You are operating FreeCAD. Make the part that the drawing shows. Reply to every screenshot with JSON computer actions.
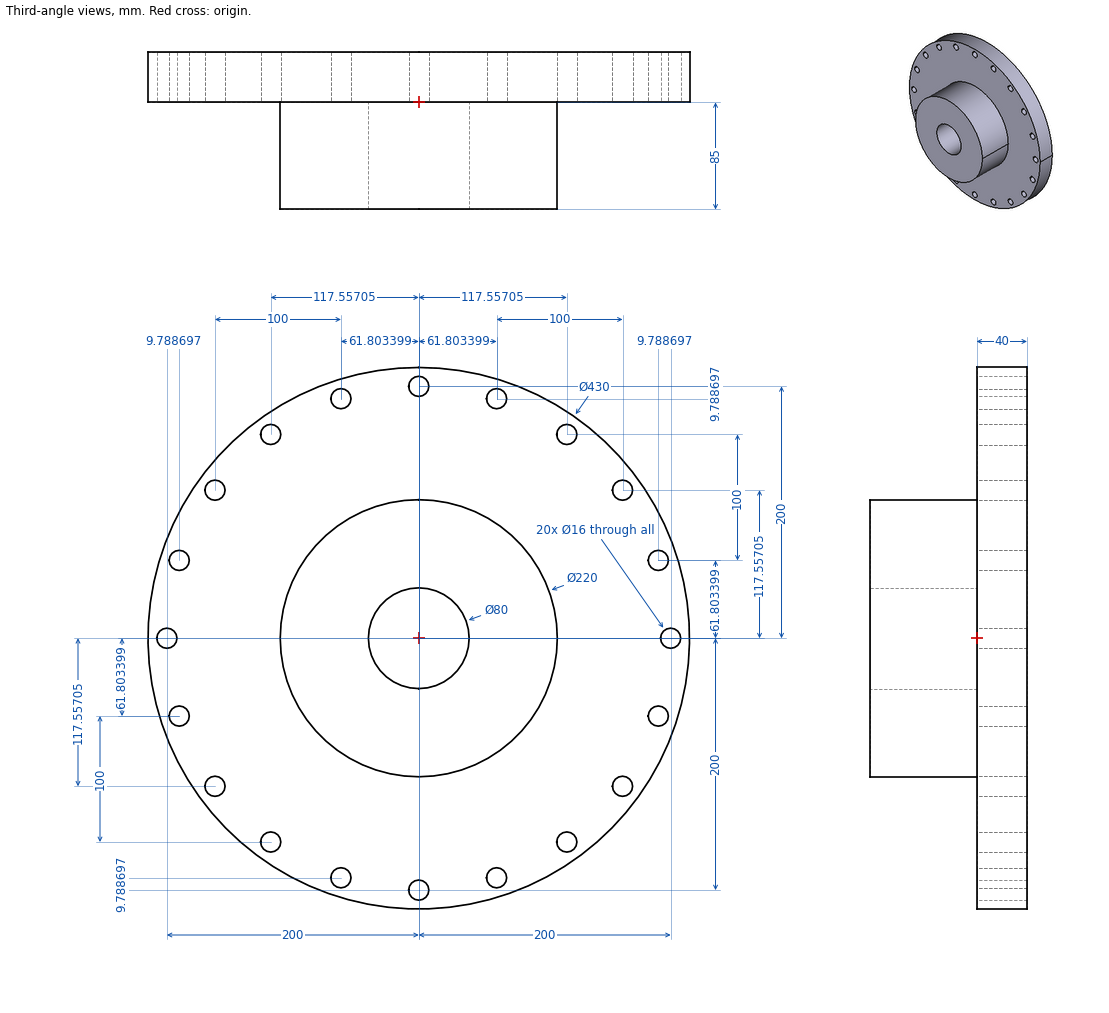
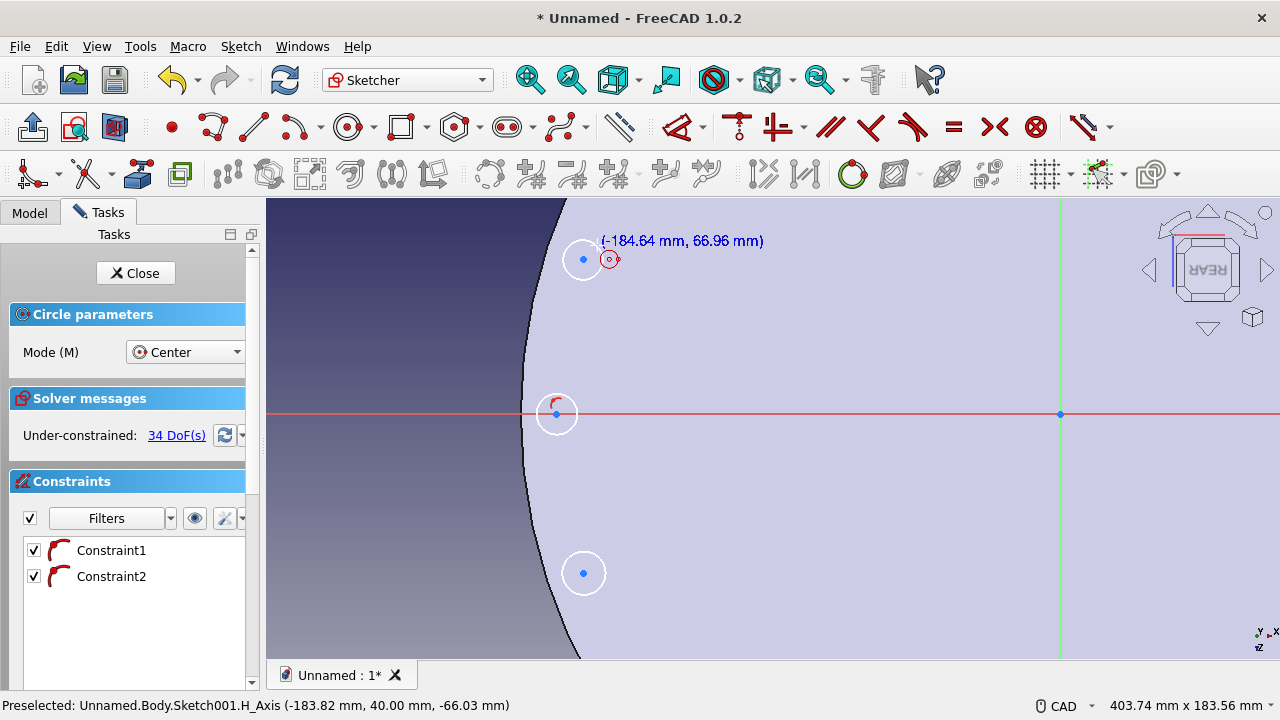
{"action": "scroll", "coordinate": [551, 435], "scroll_direction": "down", "scroll_amount": 6}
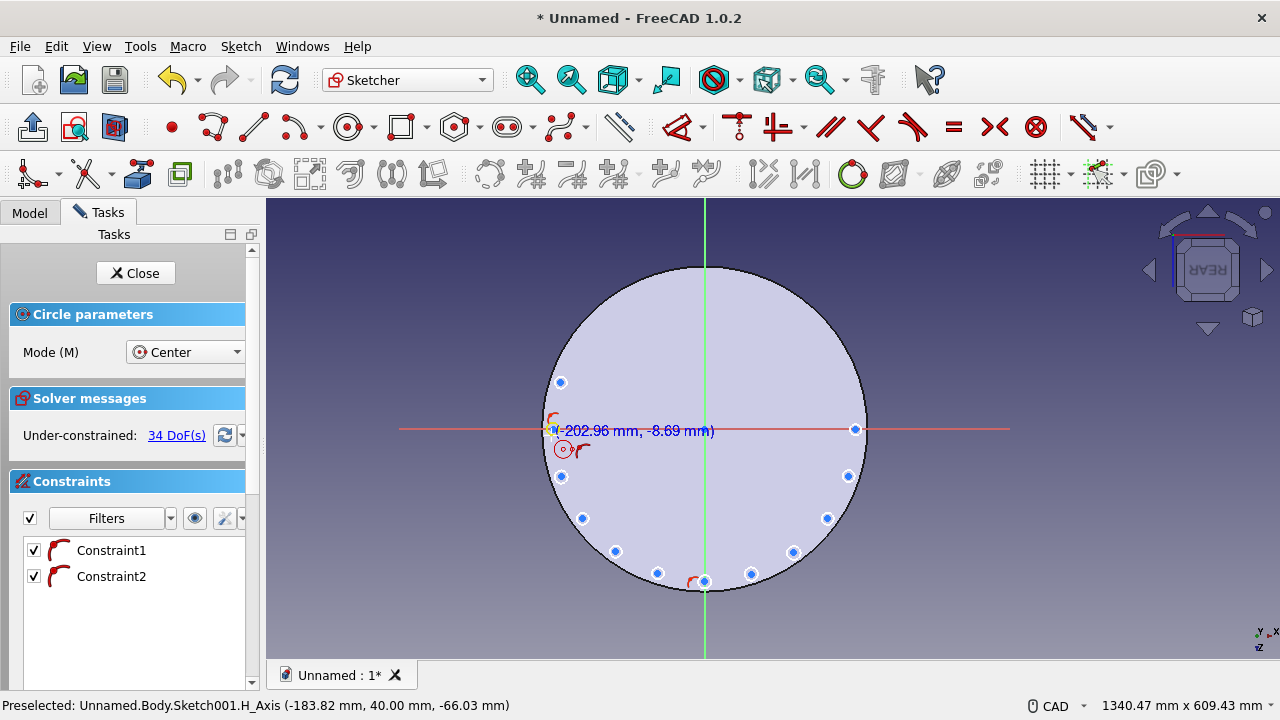
{"action": "scroll", "coordinate": [582, 340], "scroll_direction": "up", "scroll_amount": 7}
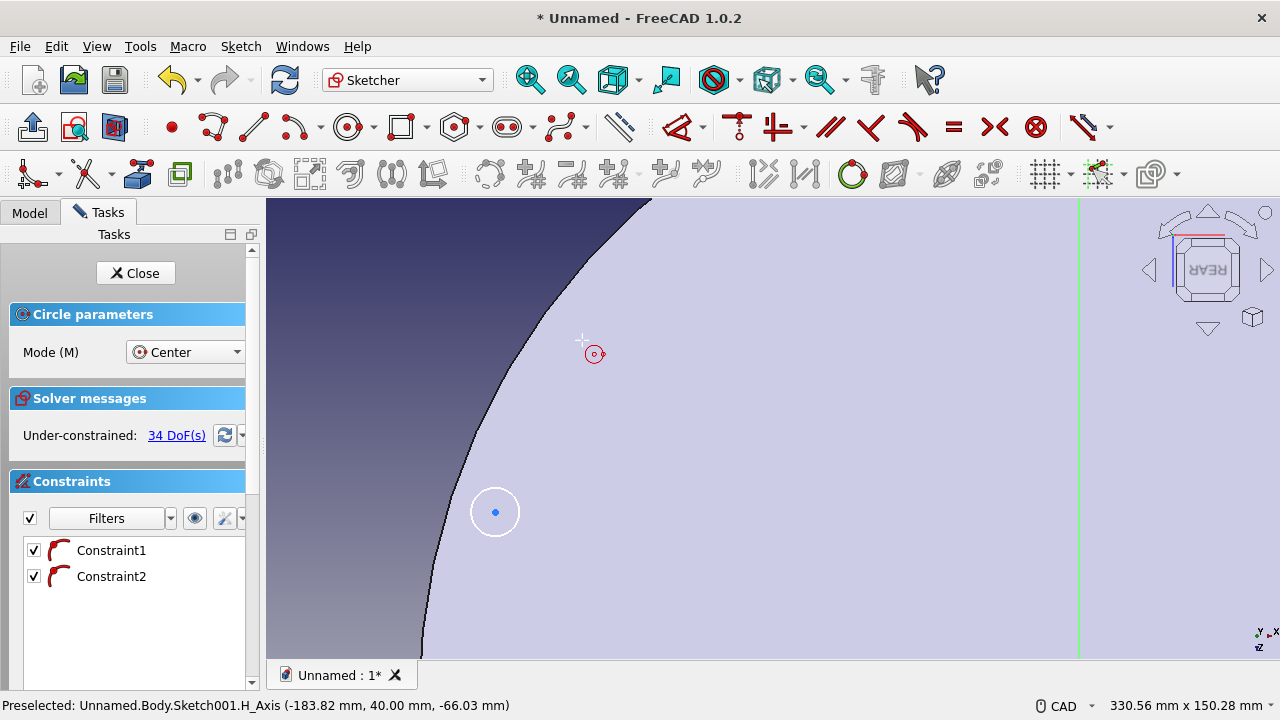
{"action": "scroll", "coordinate": [582, 340], "scroll_direction": "down", "scroll_amount": 7}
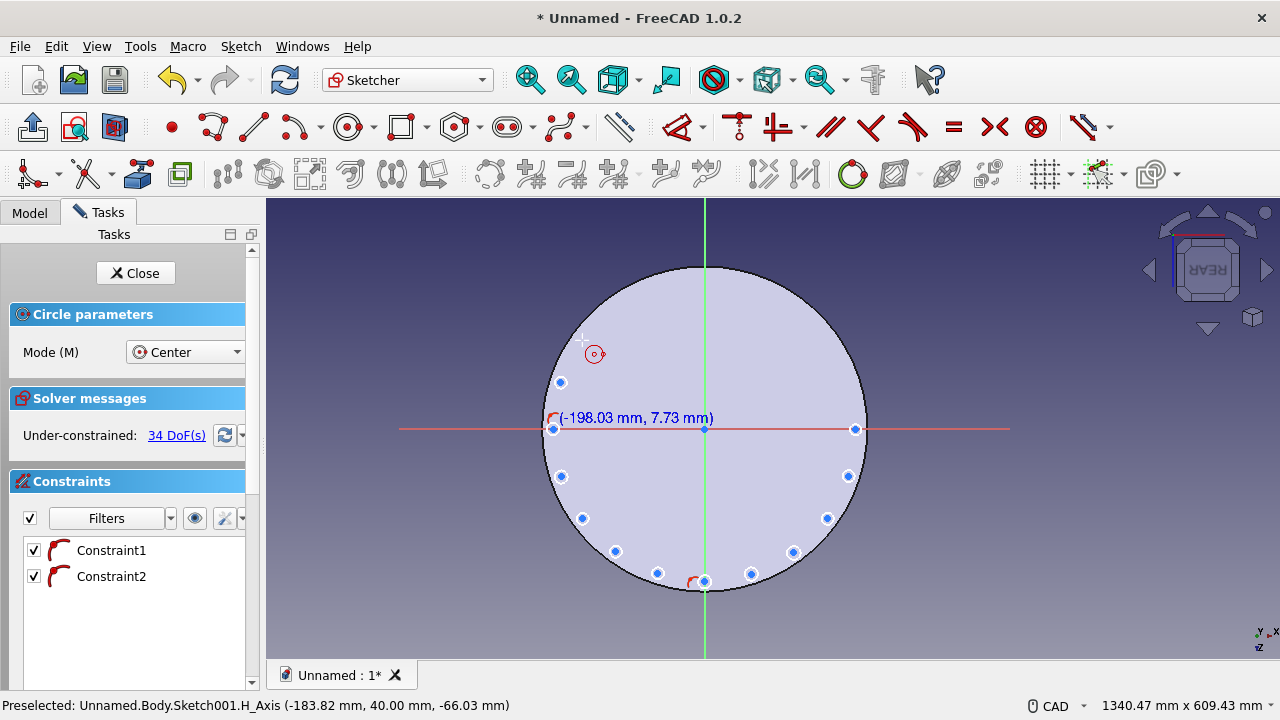
{"action": "left_click", "coordinate": [582, 340]}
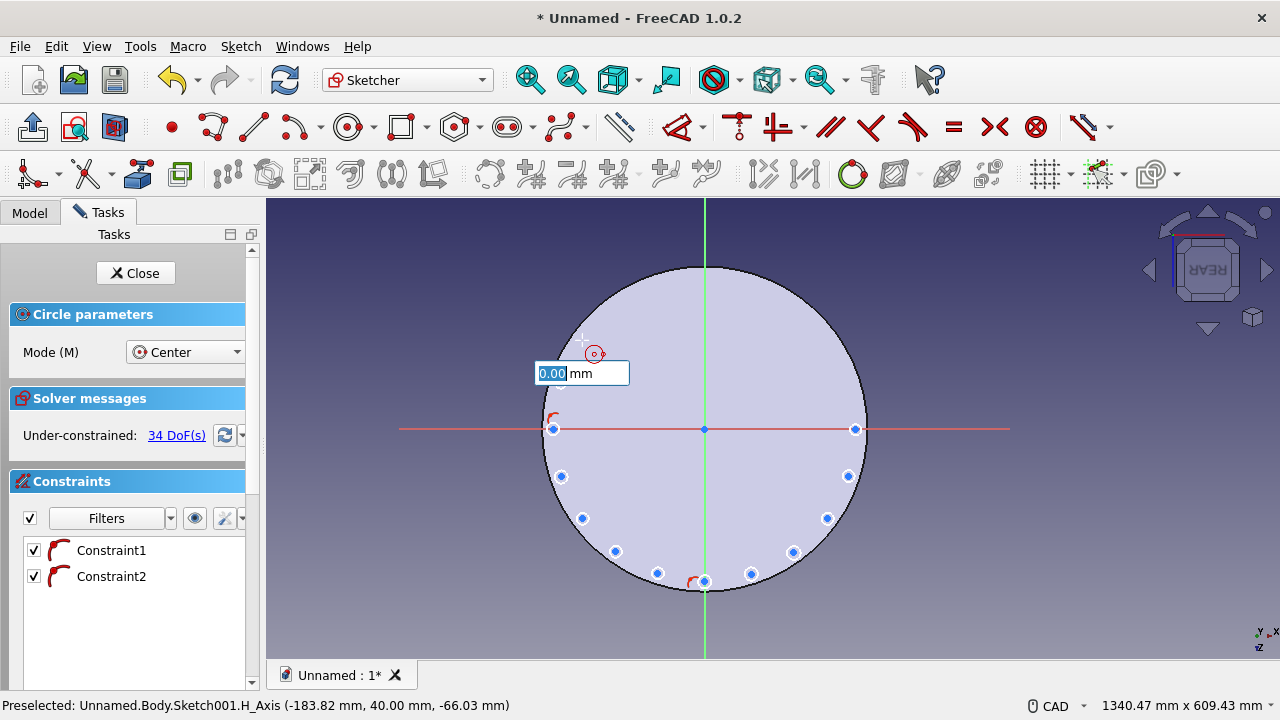
{"action": "scroll", "coordinate": [587, 336], "scroll_direction": "up", "scroll_amount": 5}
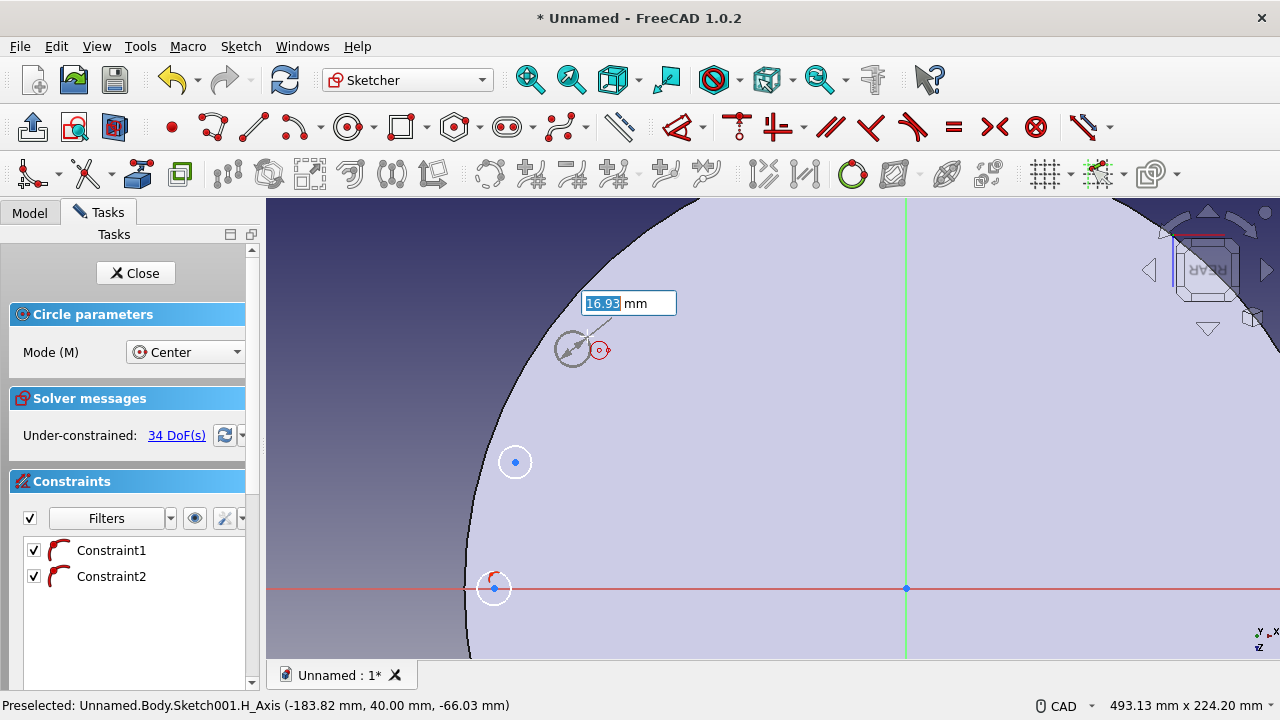
{"action": "left_click", "coordinate": [585, 335]}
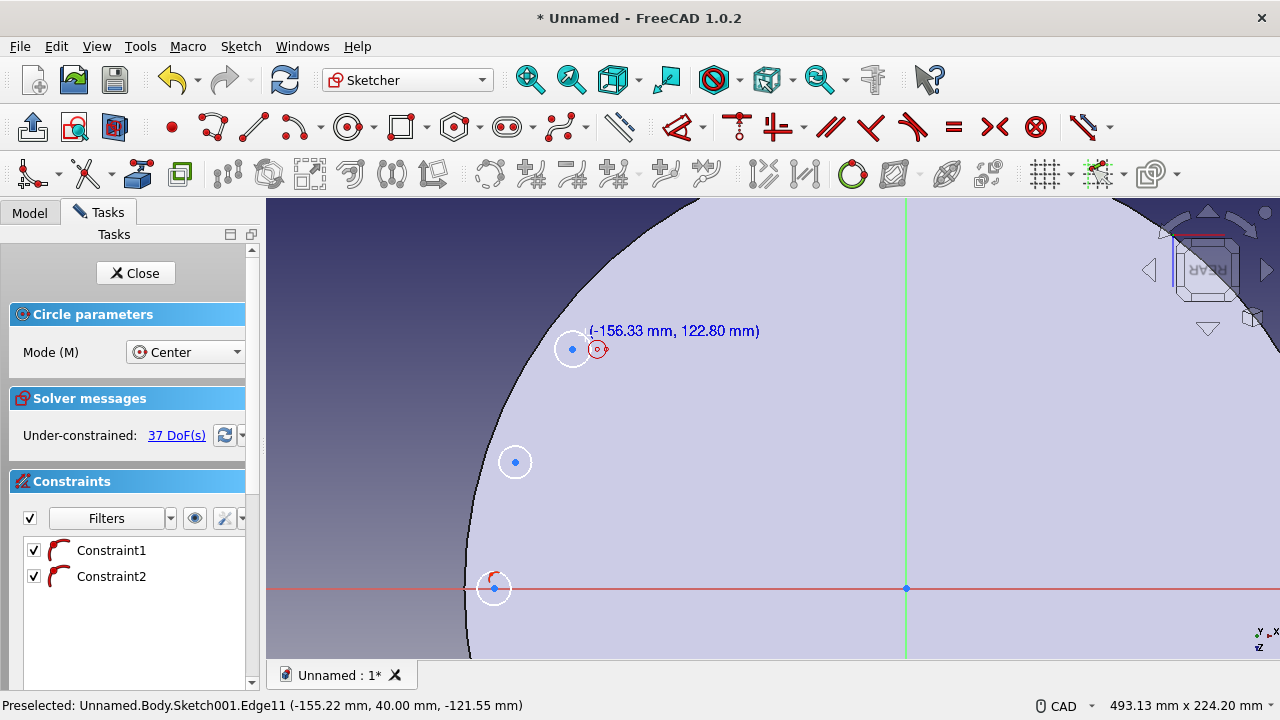
{"action": "scroll", "coordinate": [665, 256], "scroll_direction": "up", "scroll_amount": 2}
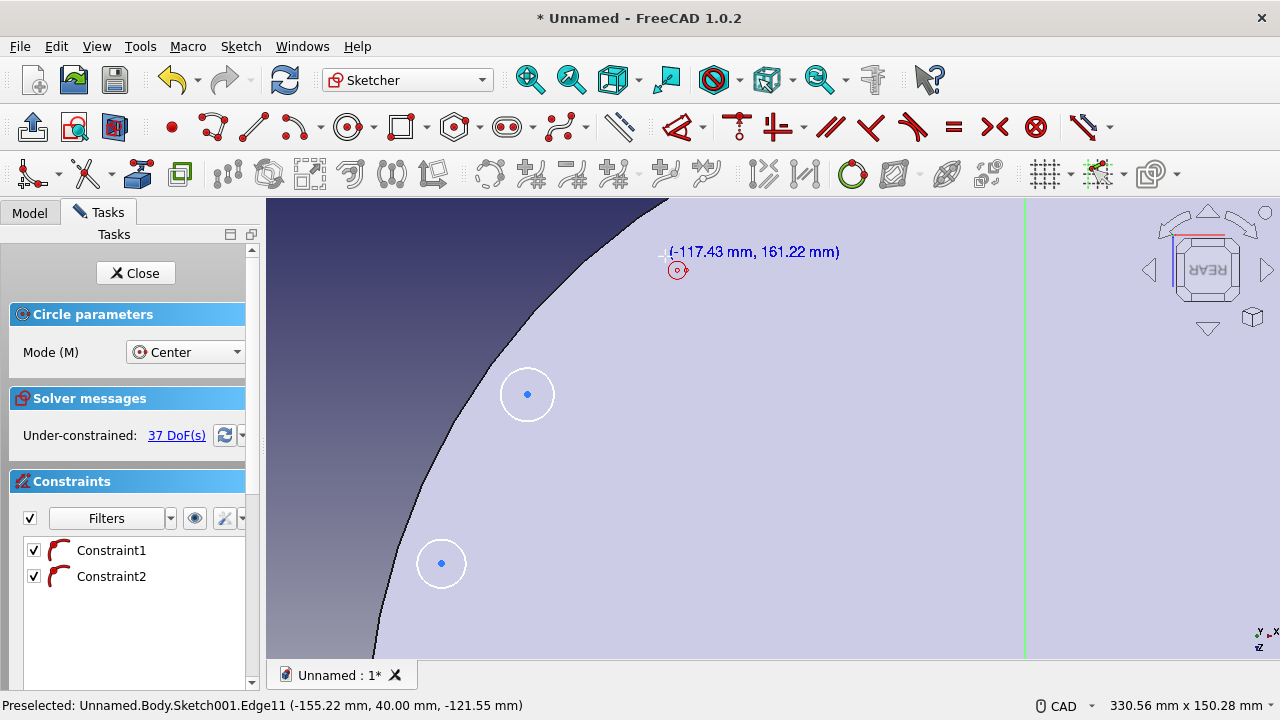
{"action": "scroll", "coordinate": [600, 323], "scroll_direction": "down", "scroll_amount": 7}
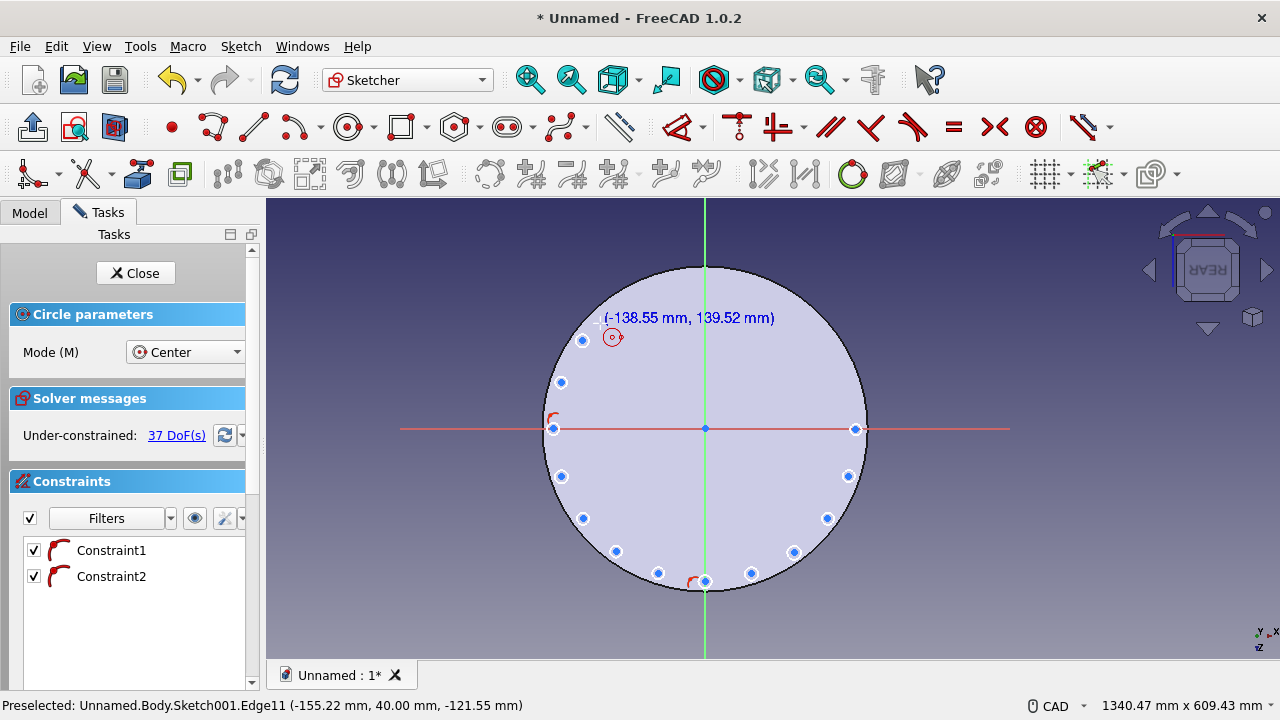
{"action": "left_click", "coordinate": [616, 307]}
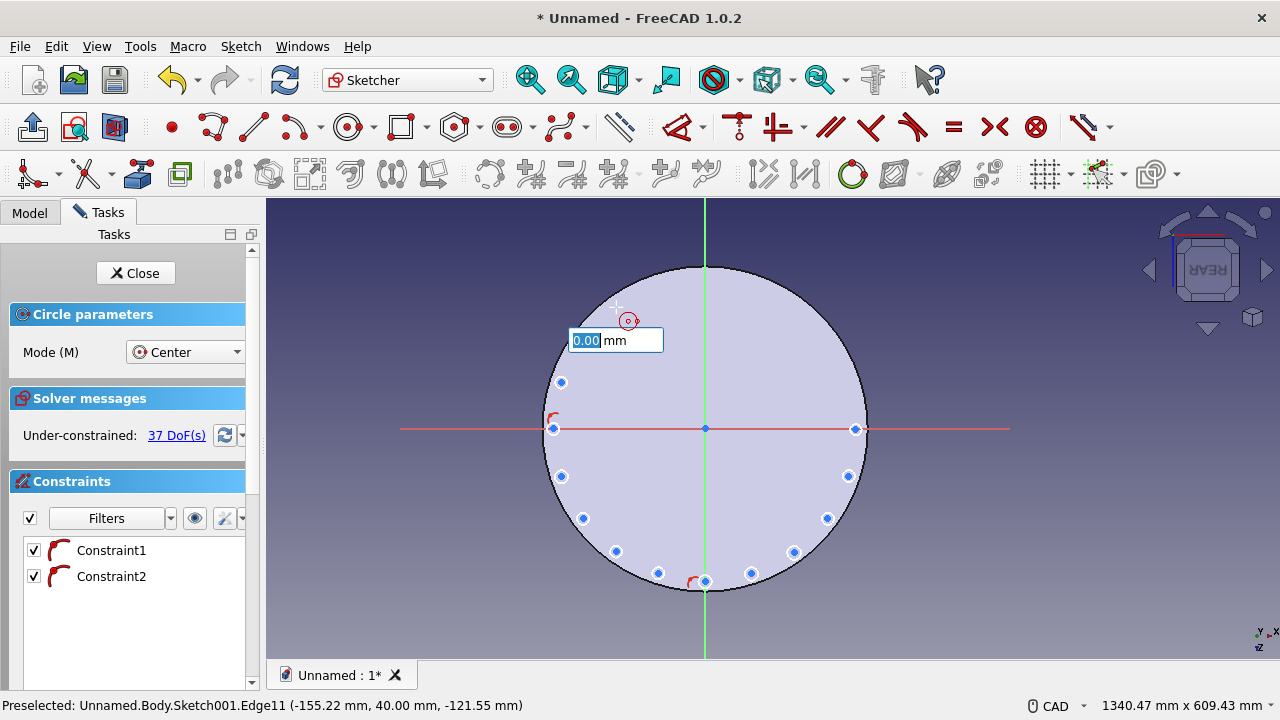
{"action": "scroll", "coordinate": [620, 302], "scroll_direction": "up", "scroll_amount": 5}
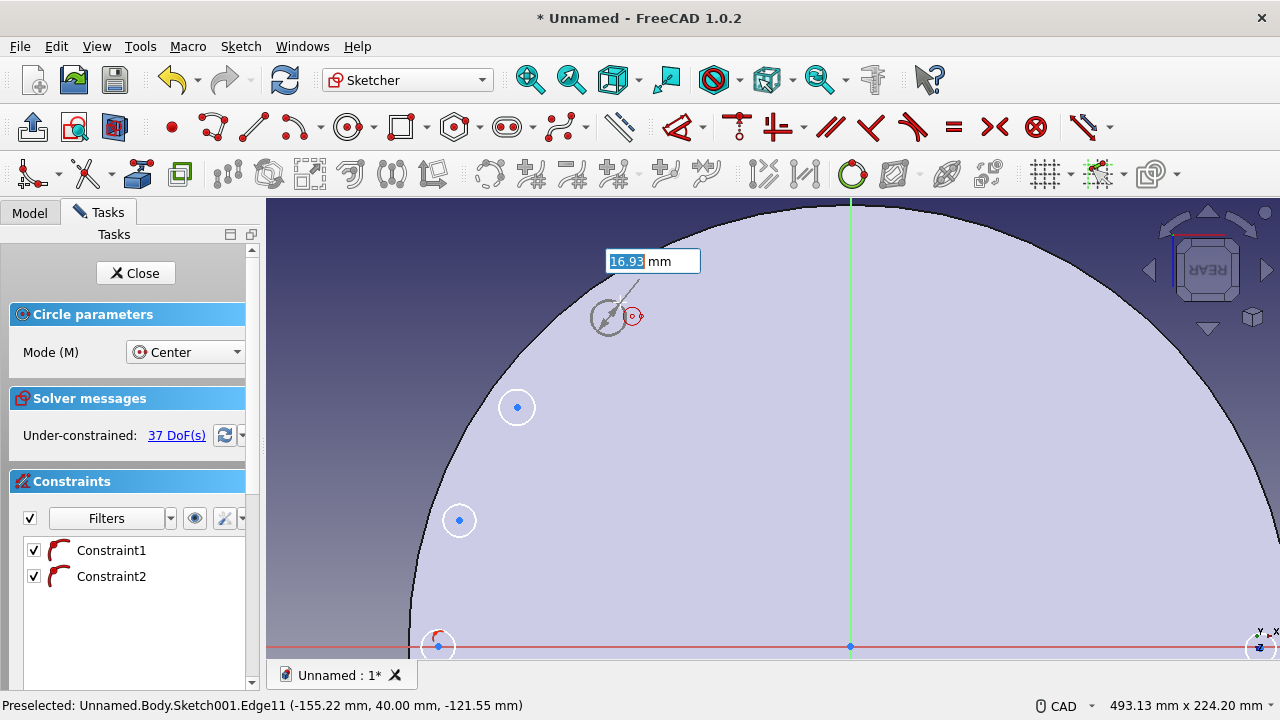
{"action": "left_click", "coordinate": [621, 302]}